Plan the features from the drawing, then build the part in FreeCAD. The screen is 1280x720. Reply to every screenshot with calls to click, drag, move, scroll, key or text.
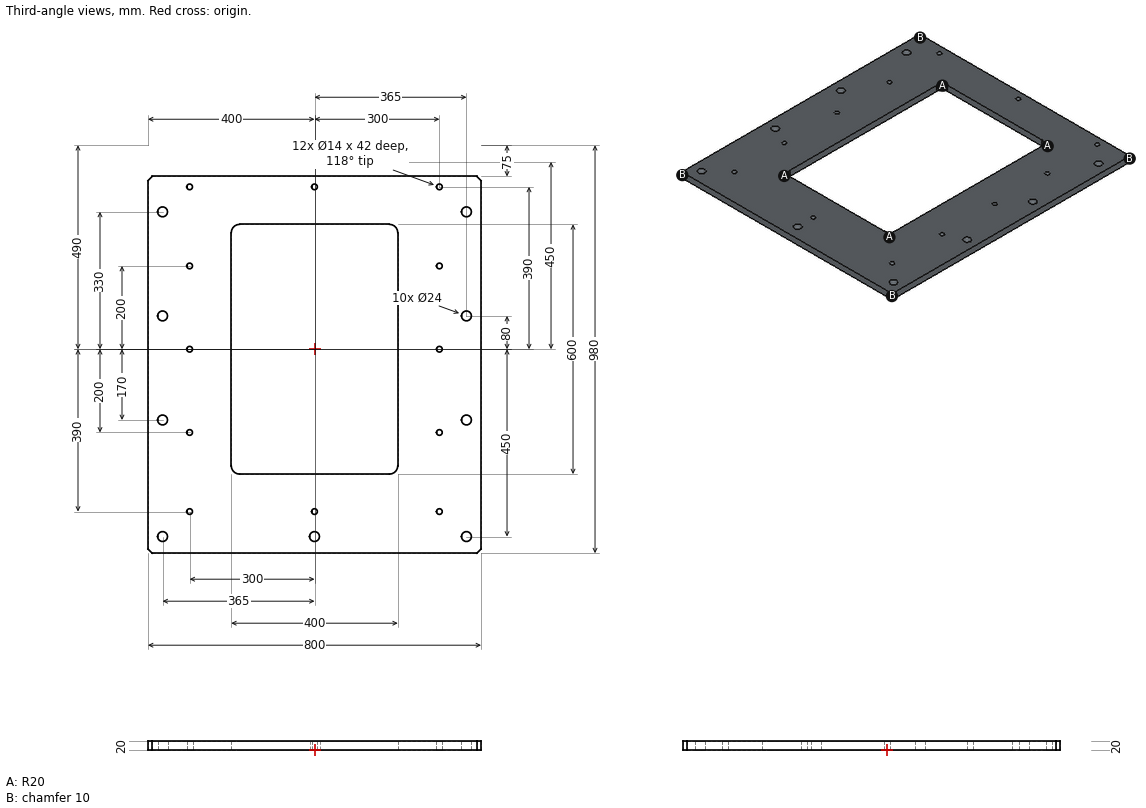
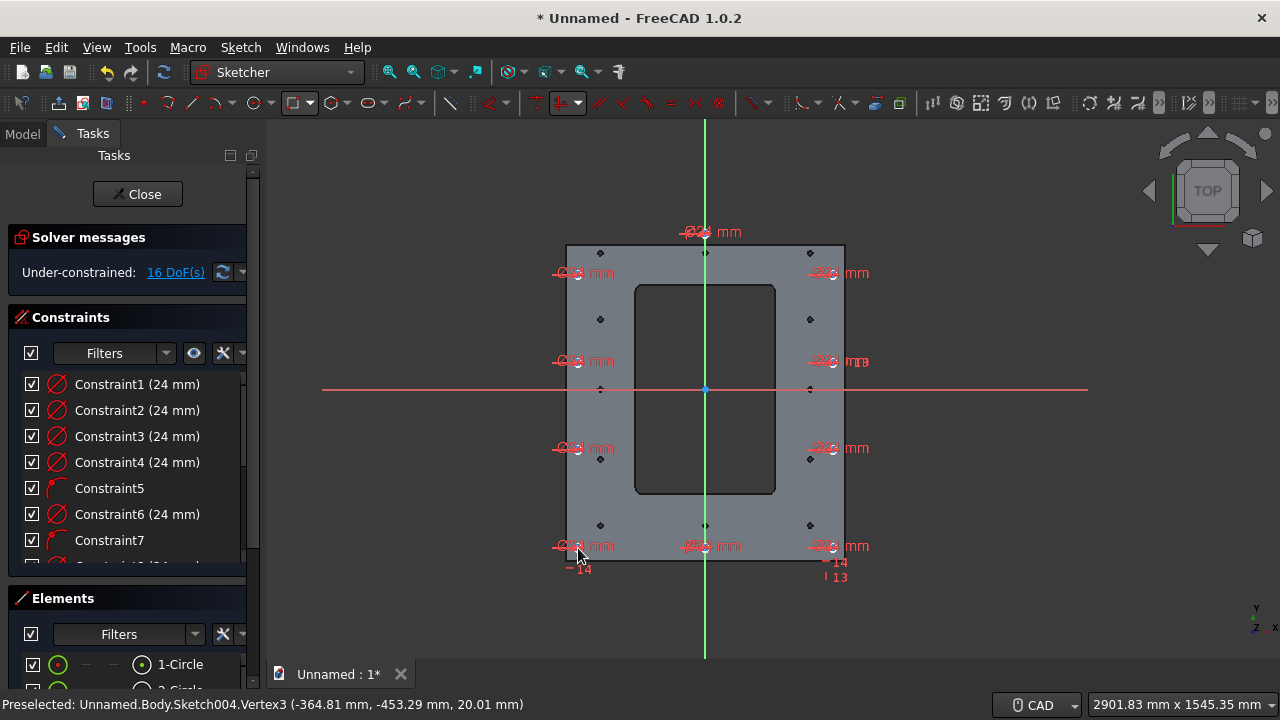
click(833, 548)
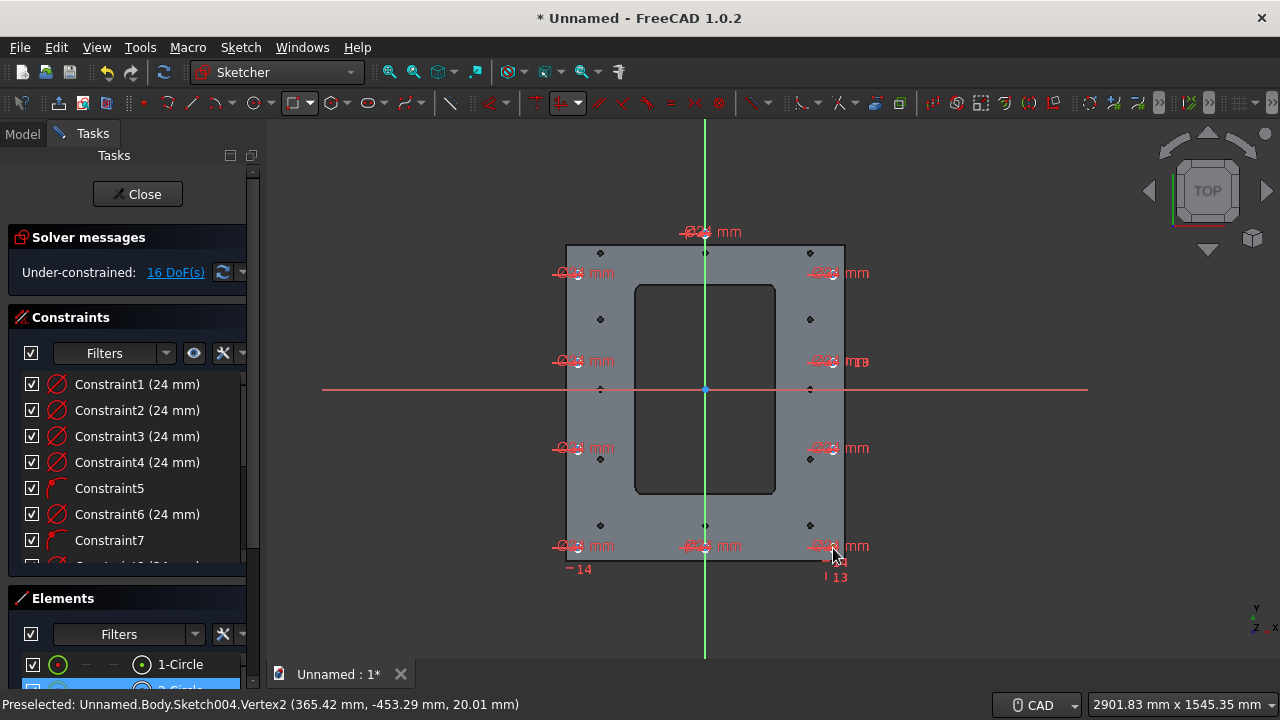
click(705, 548)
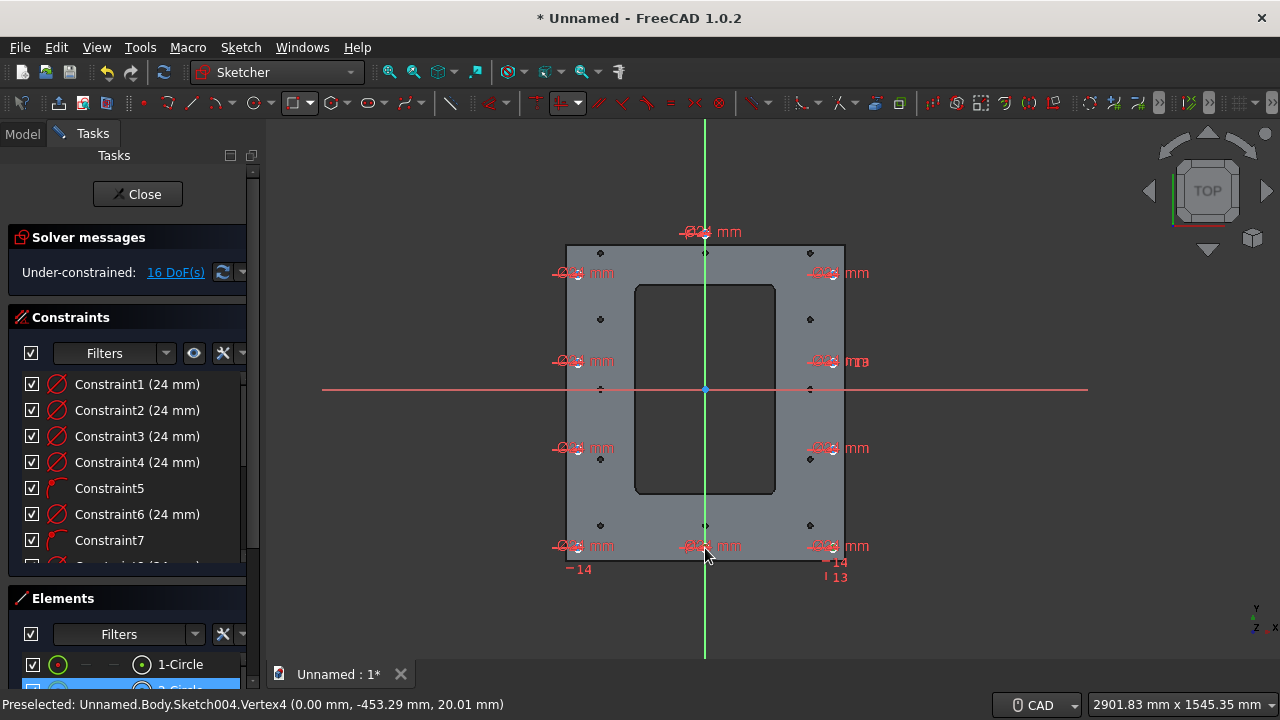
click(580, 104)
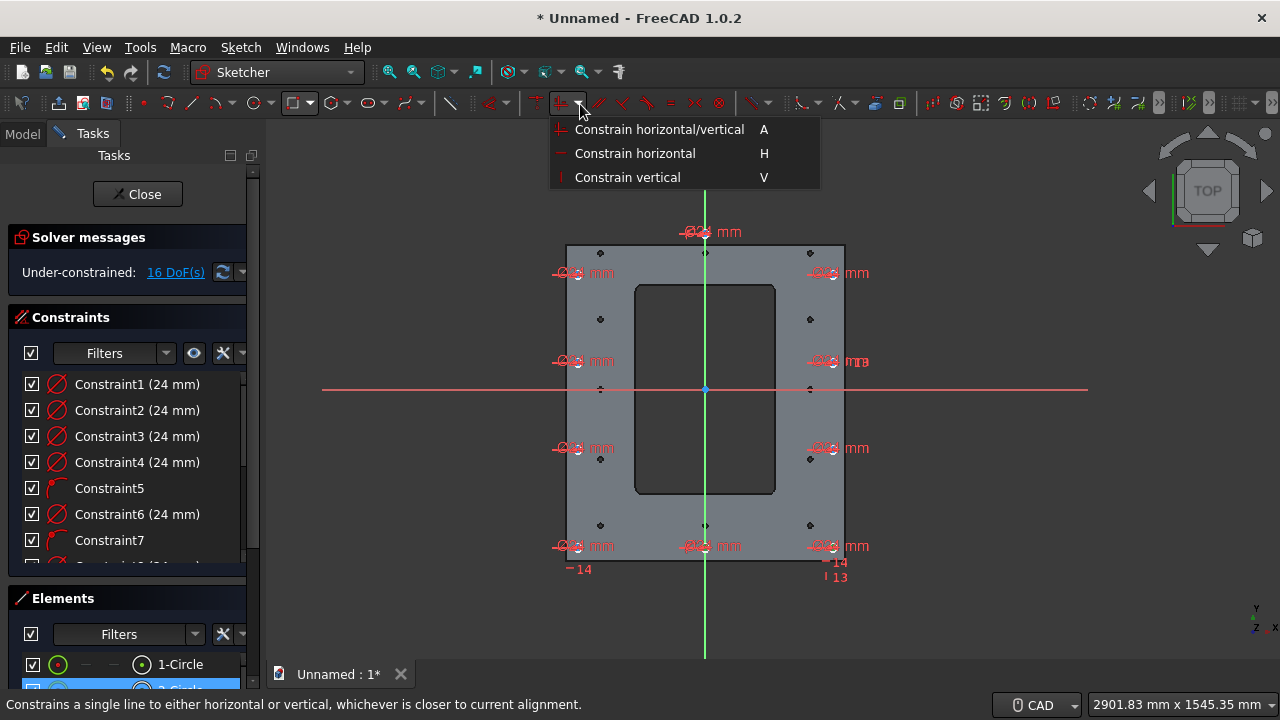
click(685, 153)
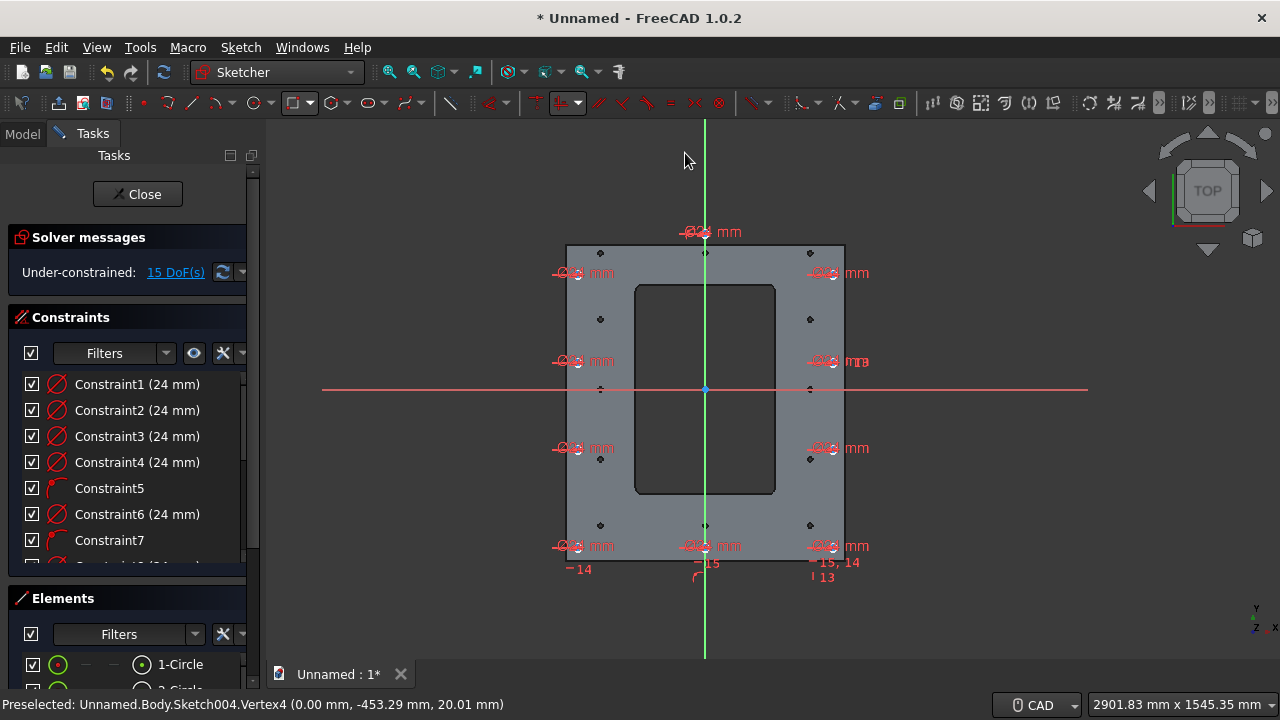
click(578, 548)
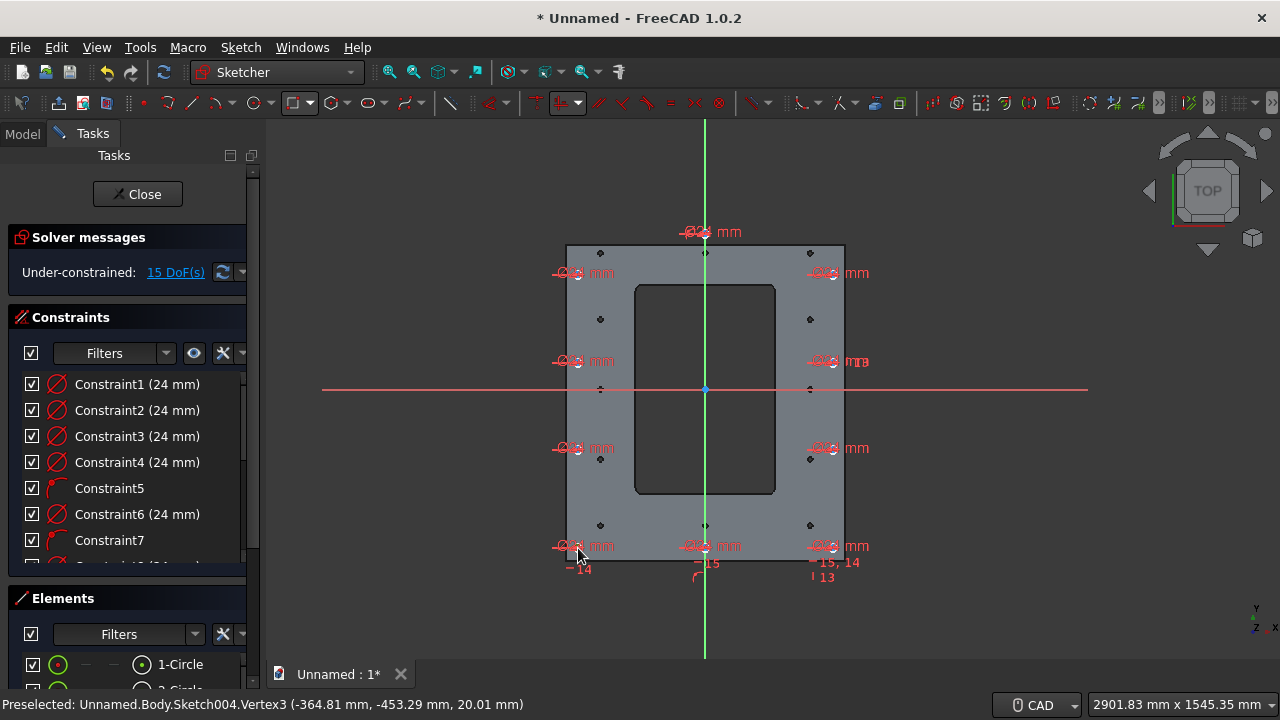
click(578, 275)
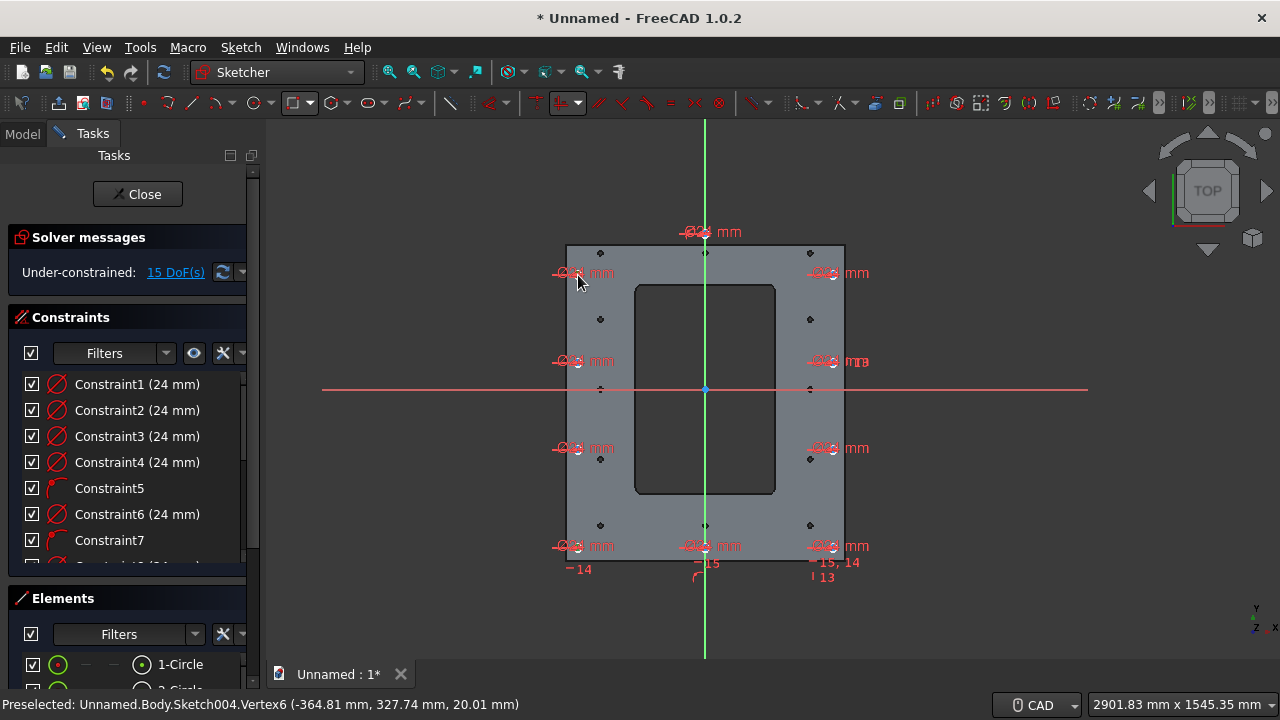
click(580, 104)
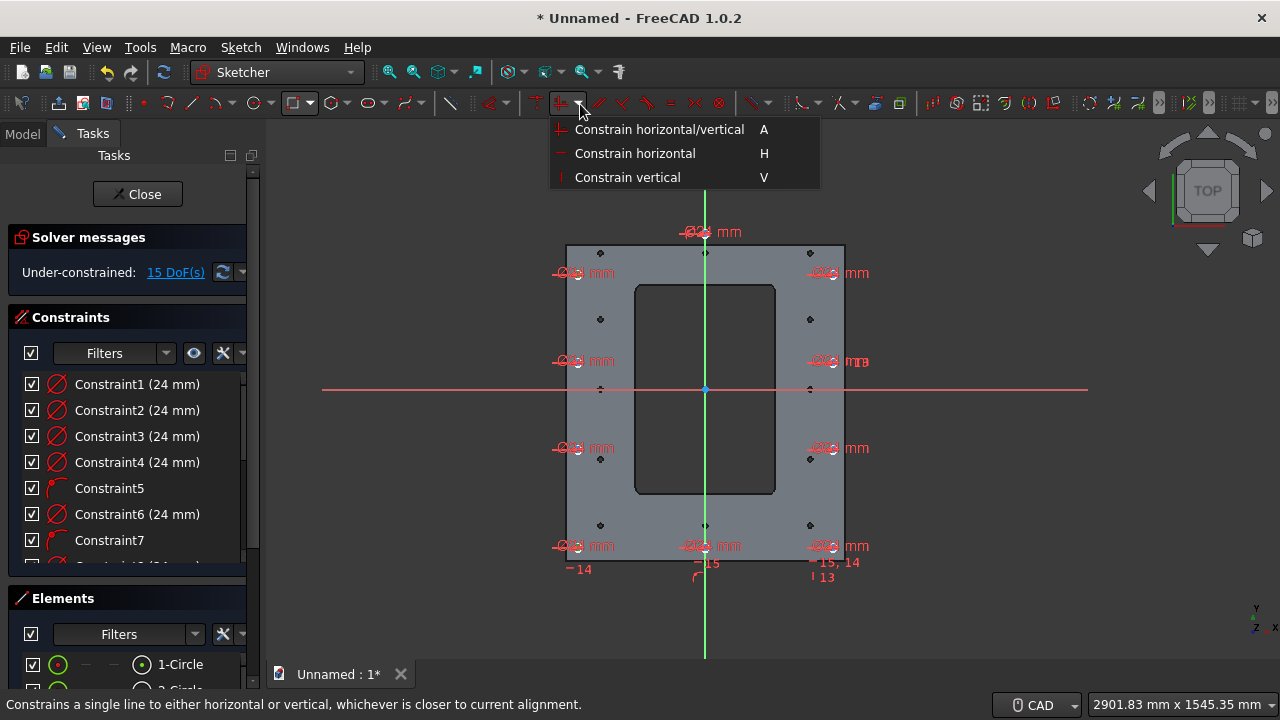
click(685, 177)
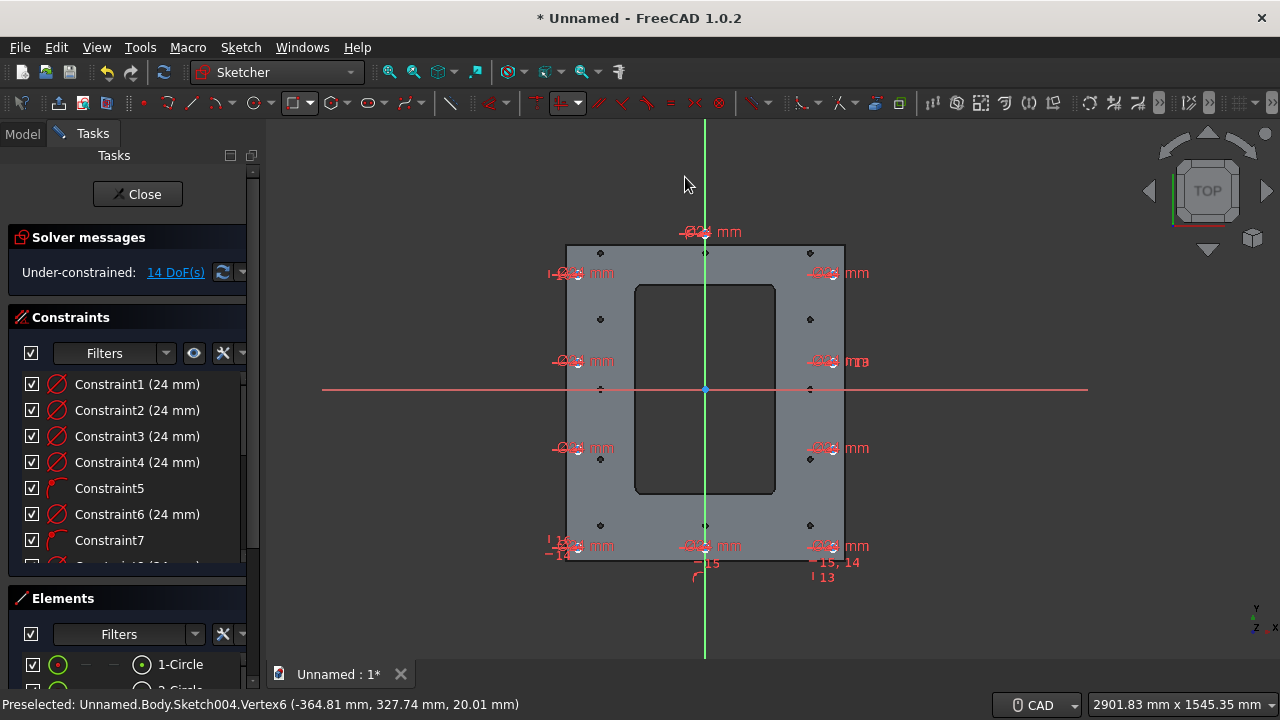
click(833, 363)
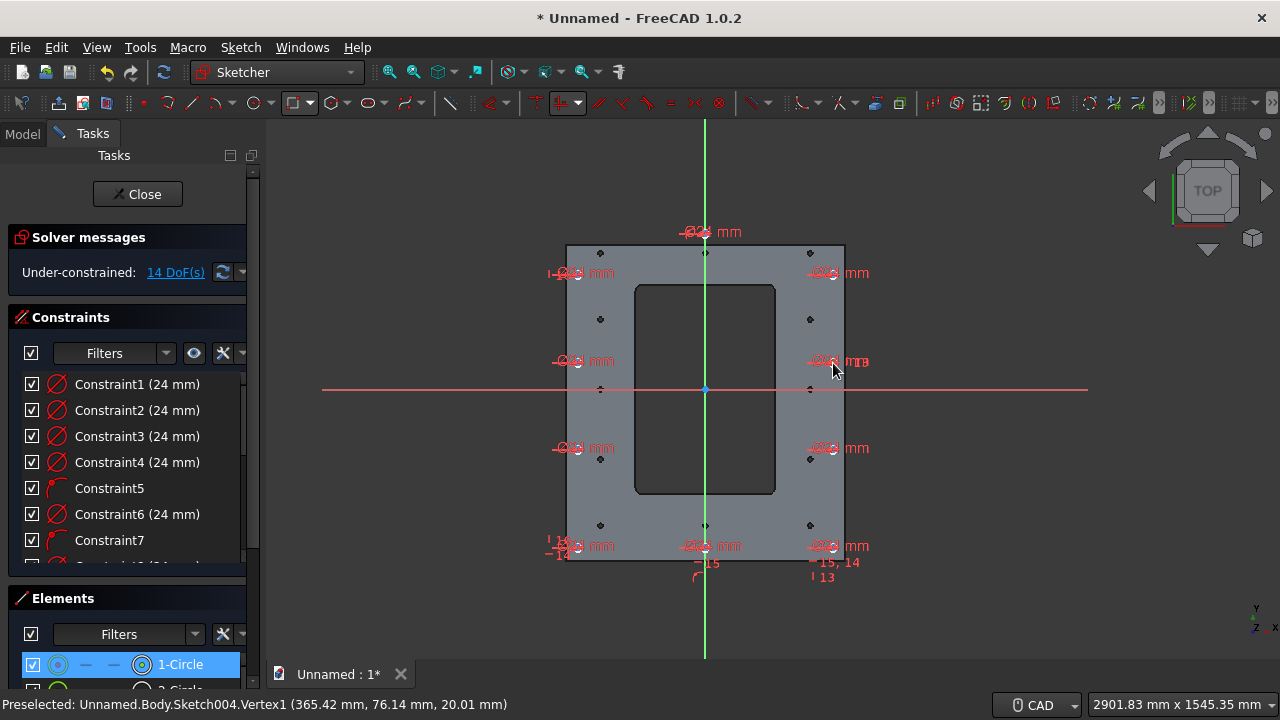
click(833, 275)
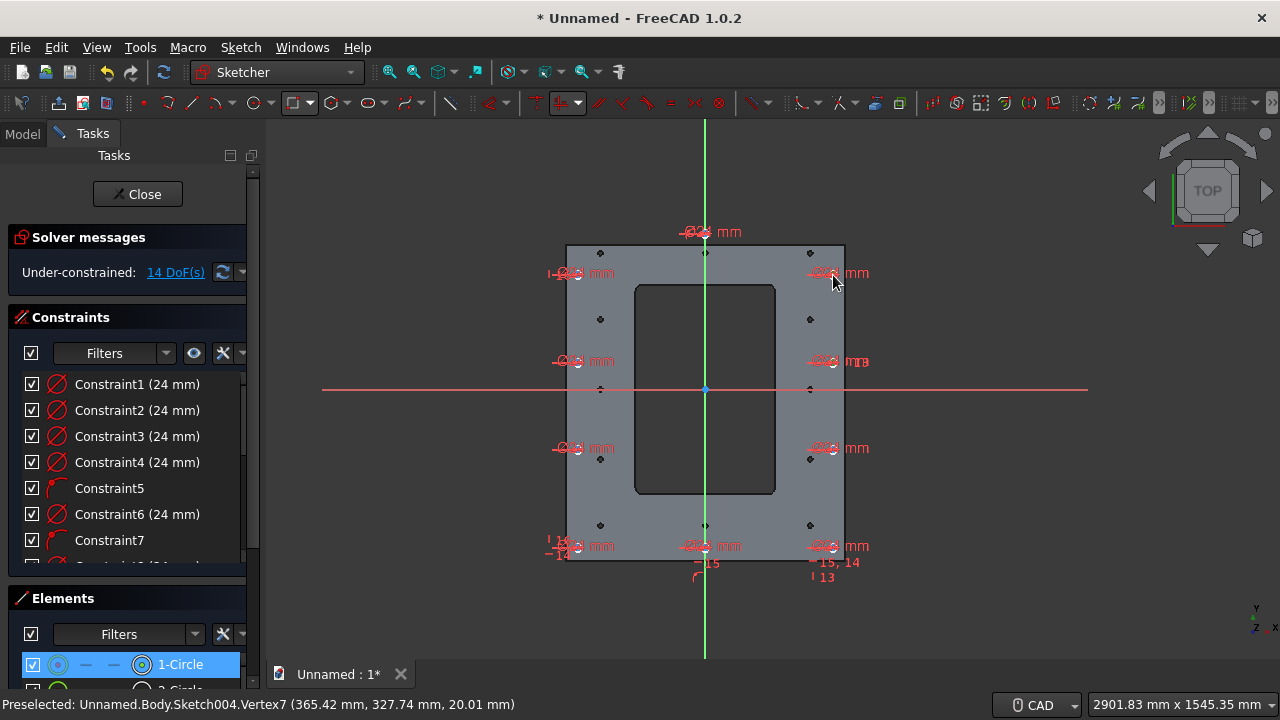
click(580, 104)